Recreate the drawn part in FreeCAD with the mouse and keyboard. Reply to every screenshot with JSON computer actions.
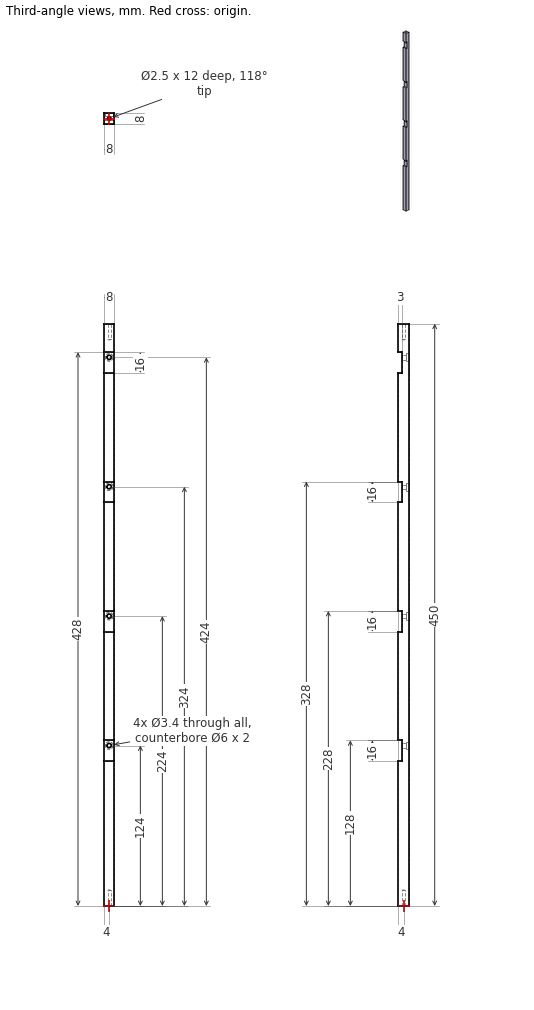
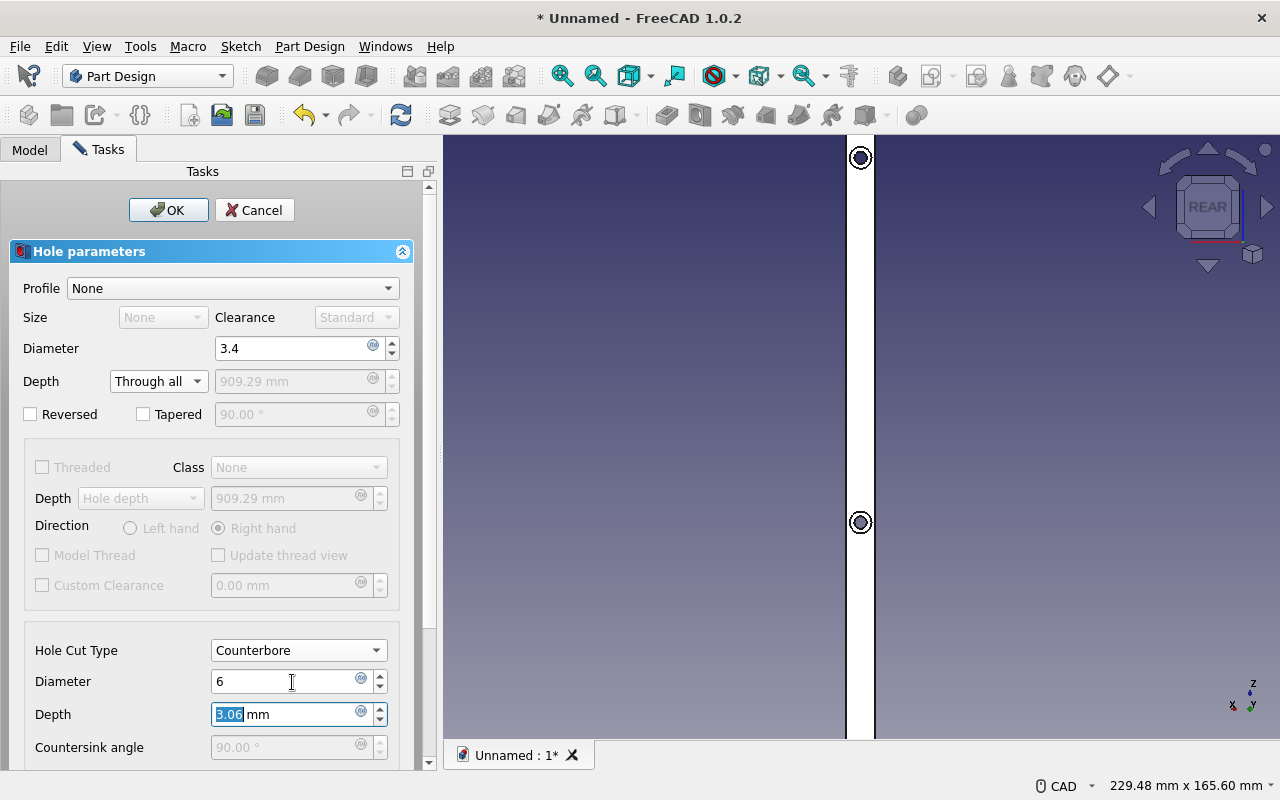
{"action": "type", "text": "2"}
{"action": "key", "text": "Tab"}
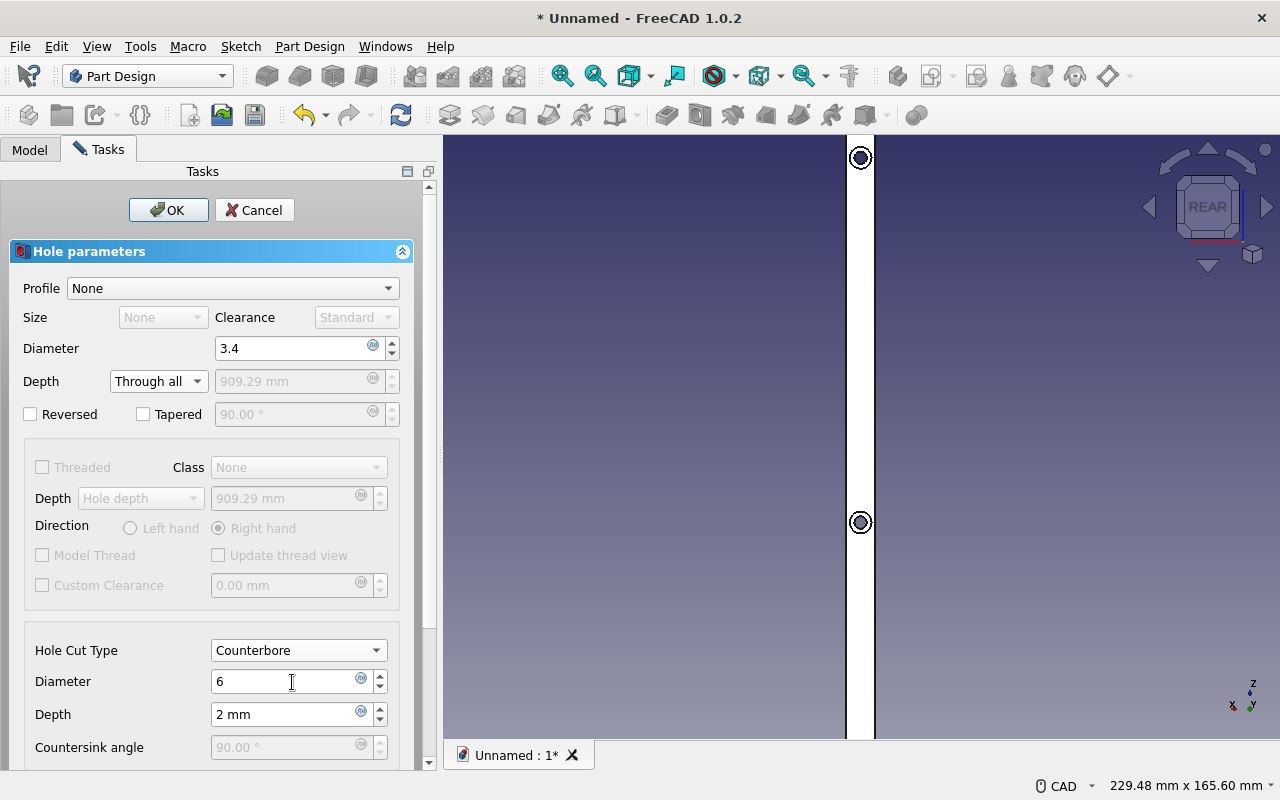
{"action": "left_click", "coordinate": [169, 210]}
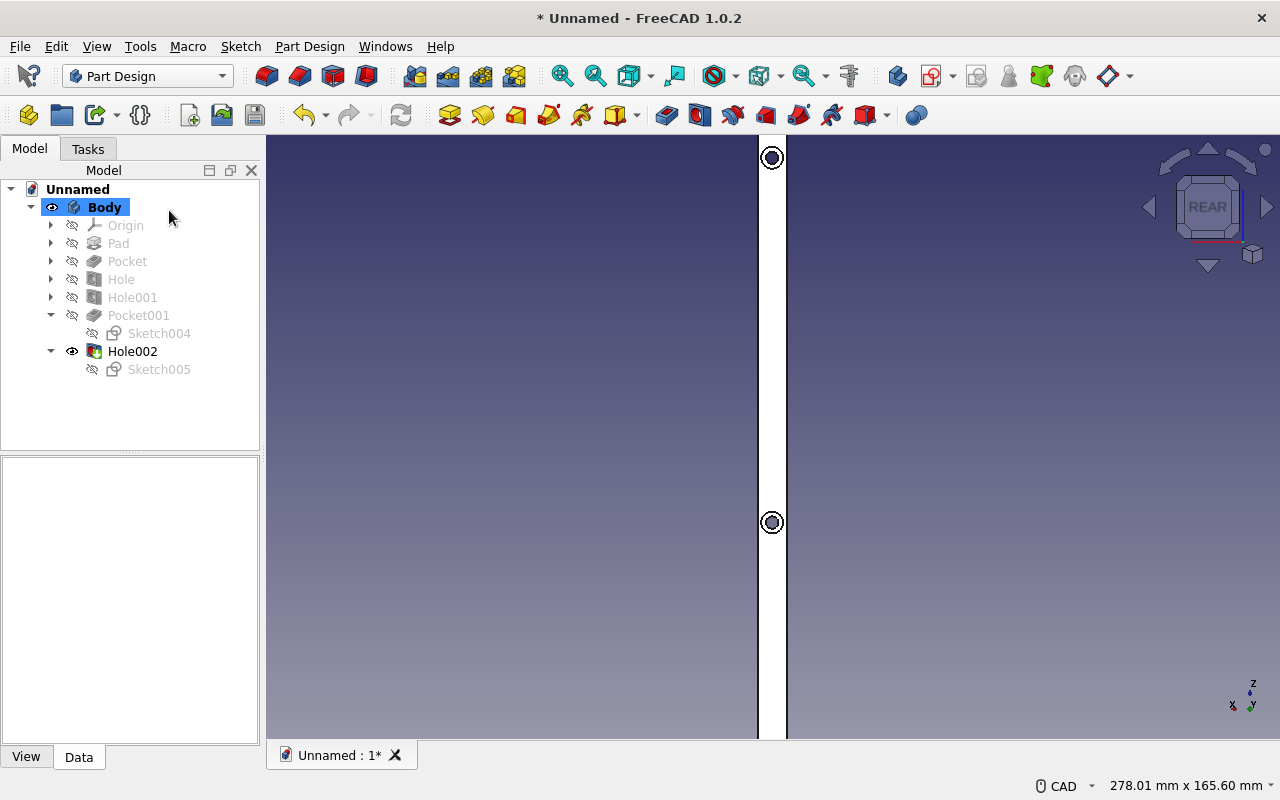
{"action": "key", "text": "0"}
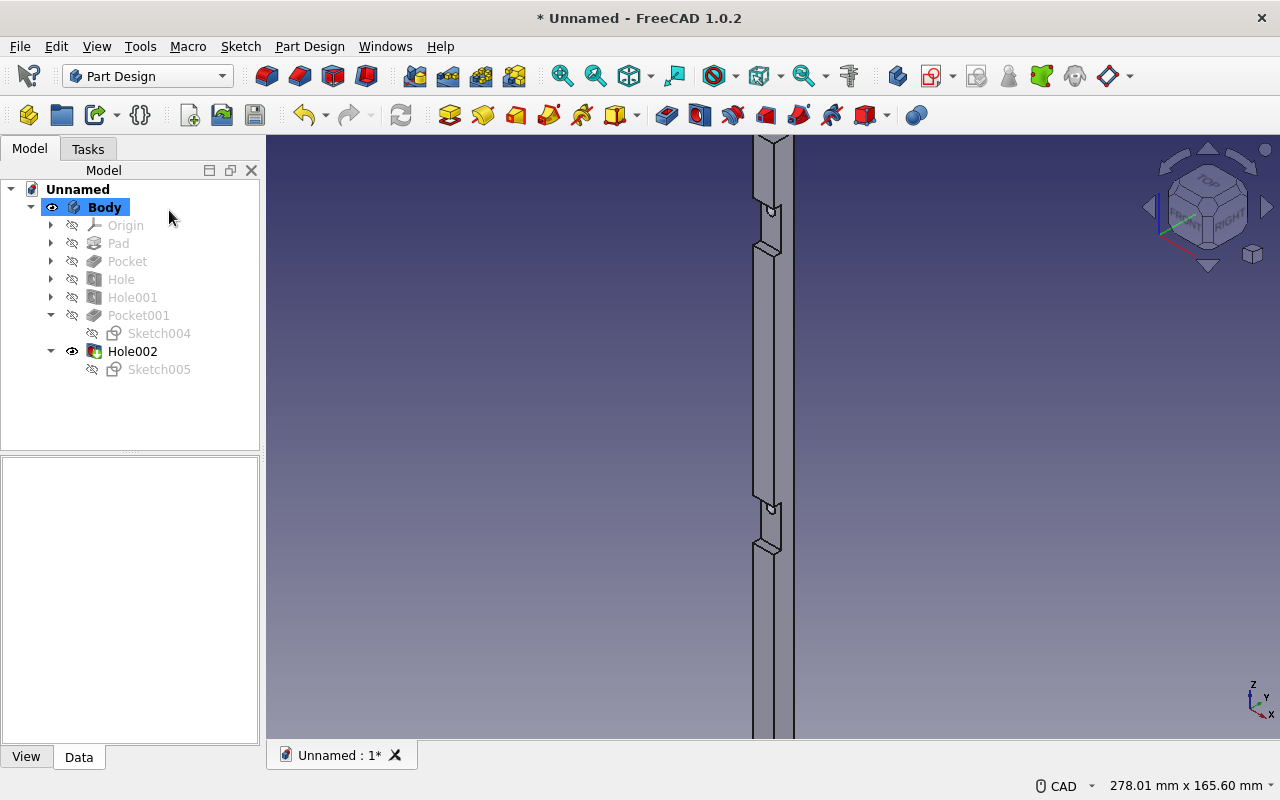
{"action": "left_click", "coordinate": [563, 76]}